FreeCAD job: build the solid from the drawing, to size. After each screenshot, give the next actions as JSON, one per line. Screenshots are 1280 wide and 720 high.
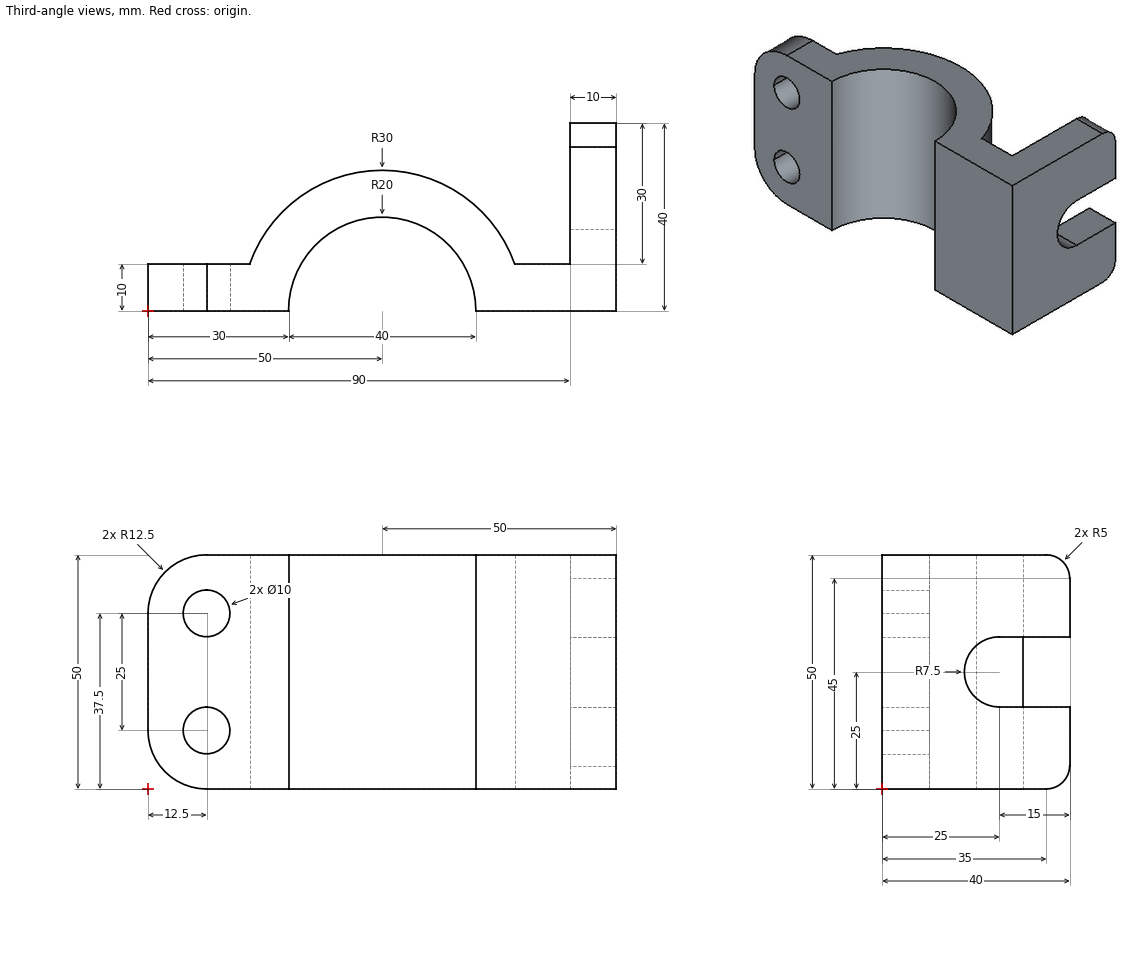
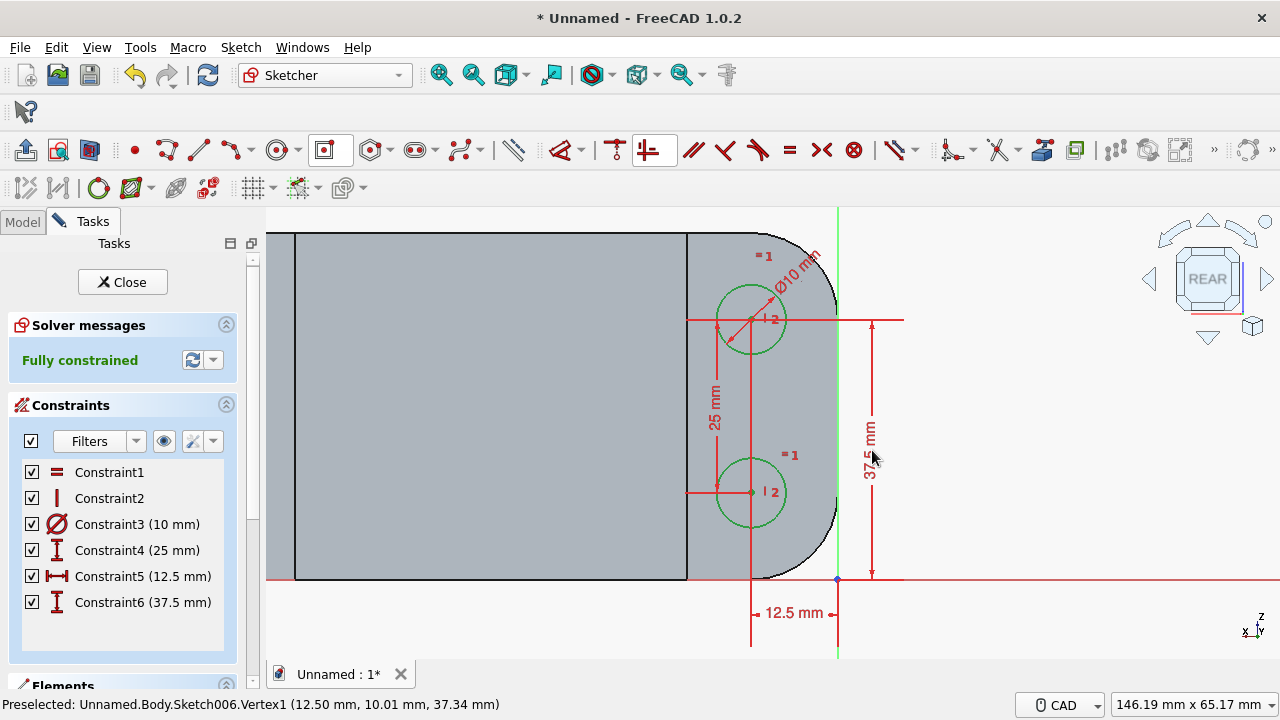
{"action": "left_click", "coordinate": [123, 282]}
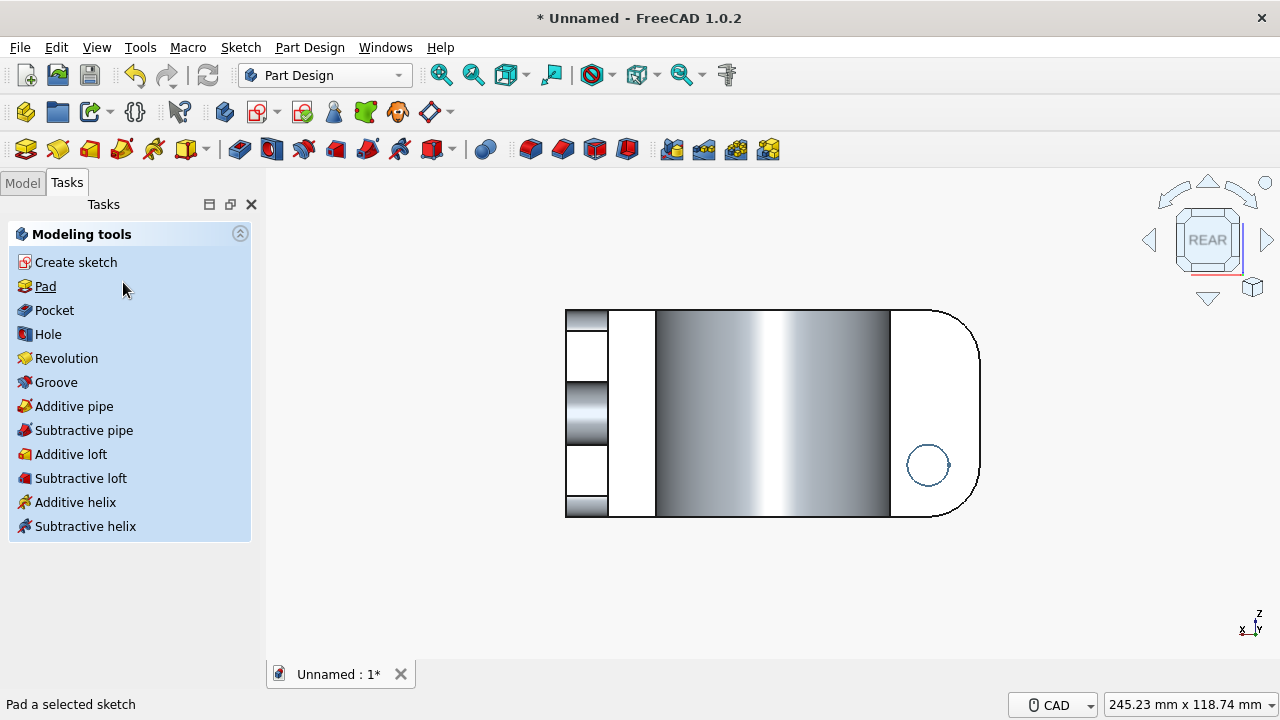
{"action": "left_click", "coordinate": [240, 150]}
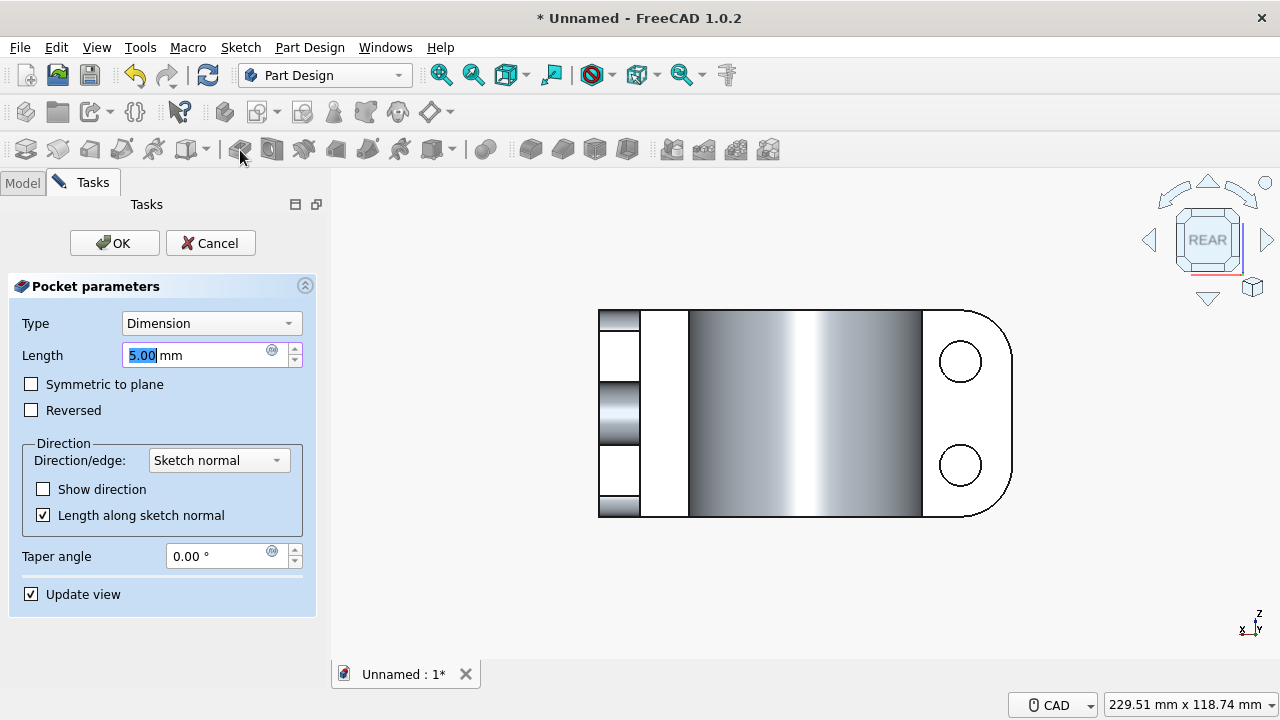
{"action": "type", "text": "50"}
{"action": "key", "text": "Tab"}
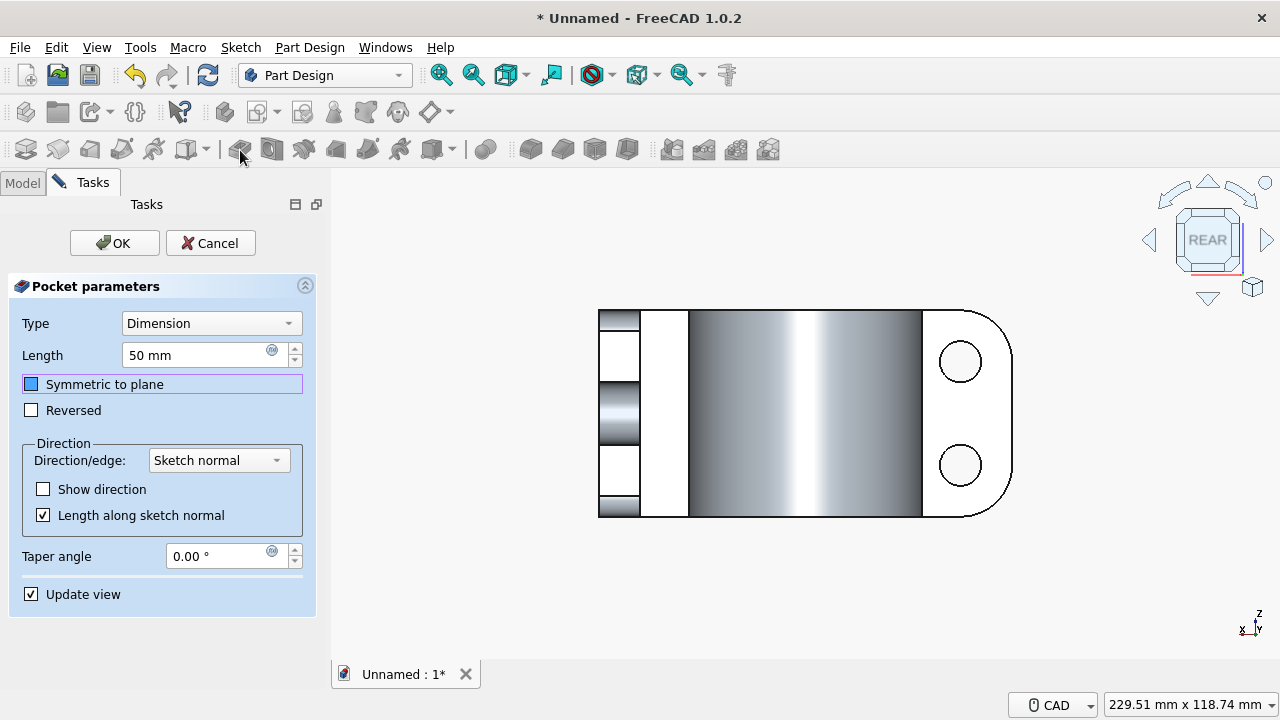
{"action": "left_click", "coordinate": [115, 243]}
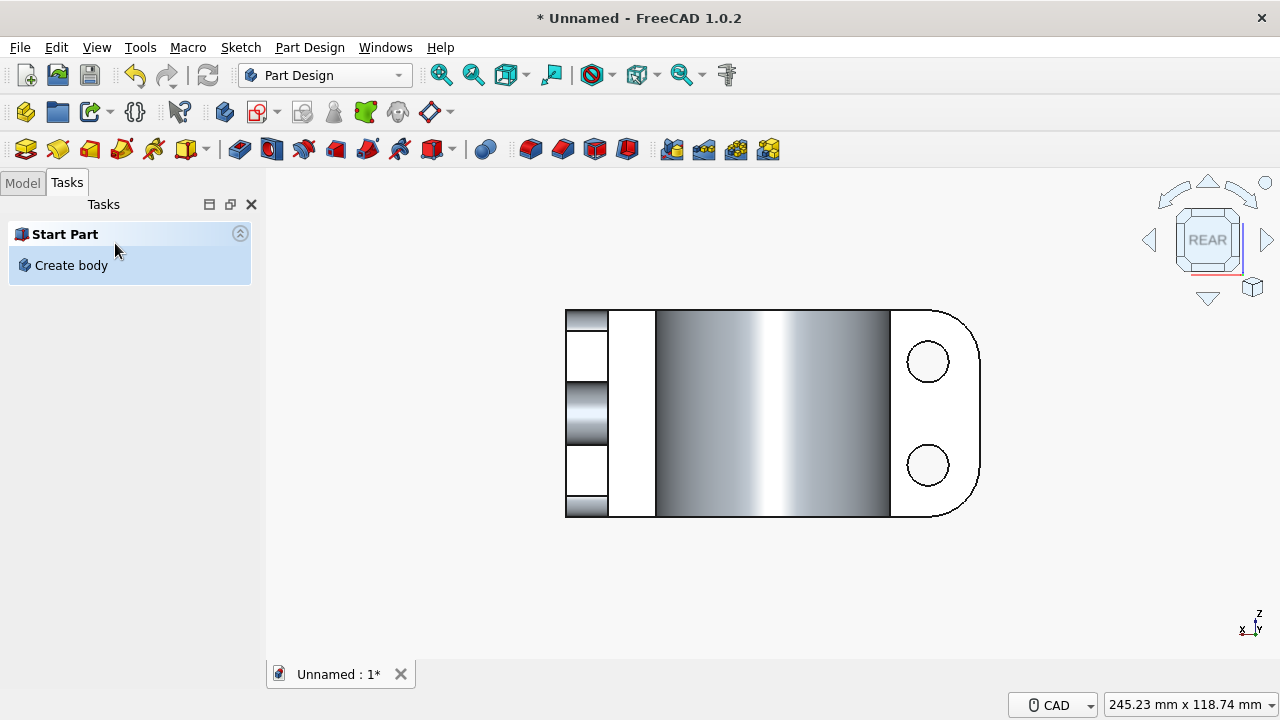
{"action": "key", "text": "0"}